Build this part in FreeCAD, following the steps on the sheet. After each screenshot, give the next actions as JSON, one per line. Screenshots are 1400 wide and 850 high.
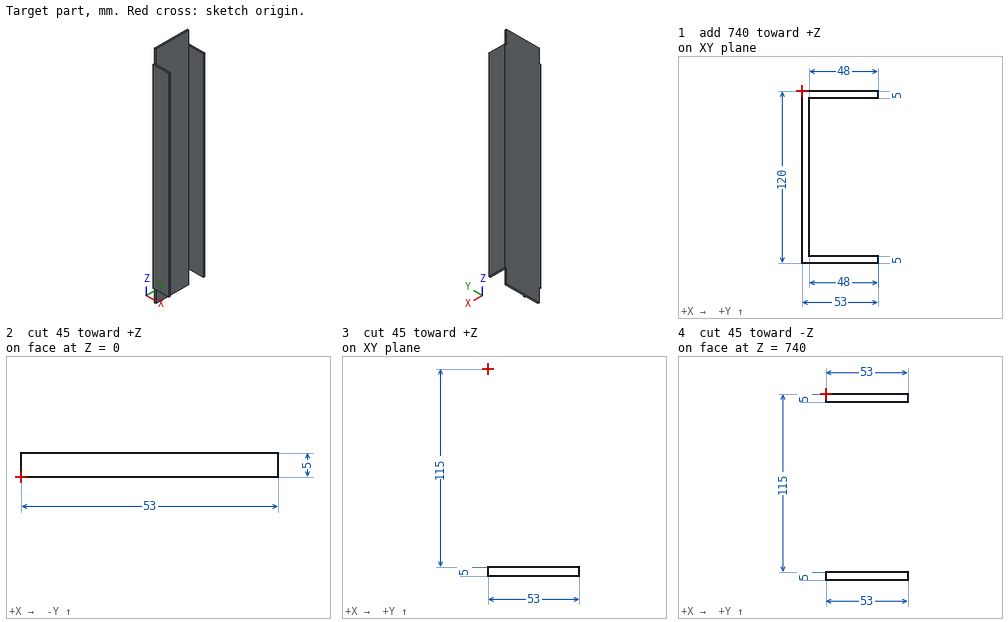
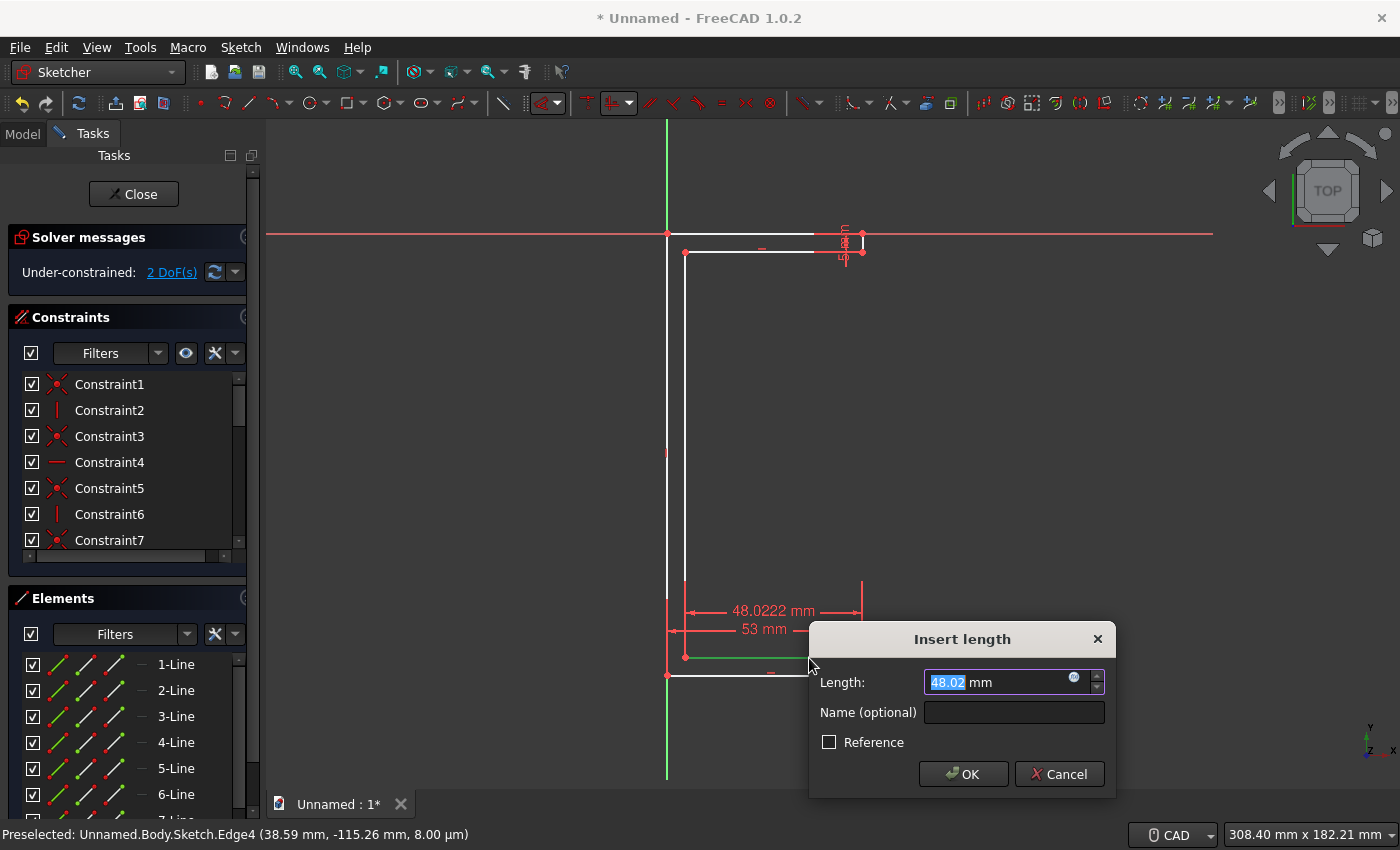
{"action": "type", "text": "48"}
{"action": "key", "text": "Return"}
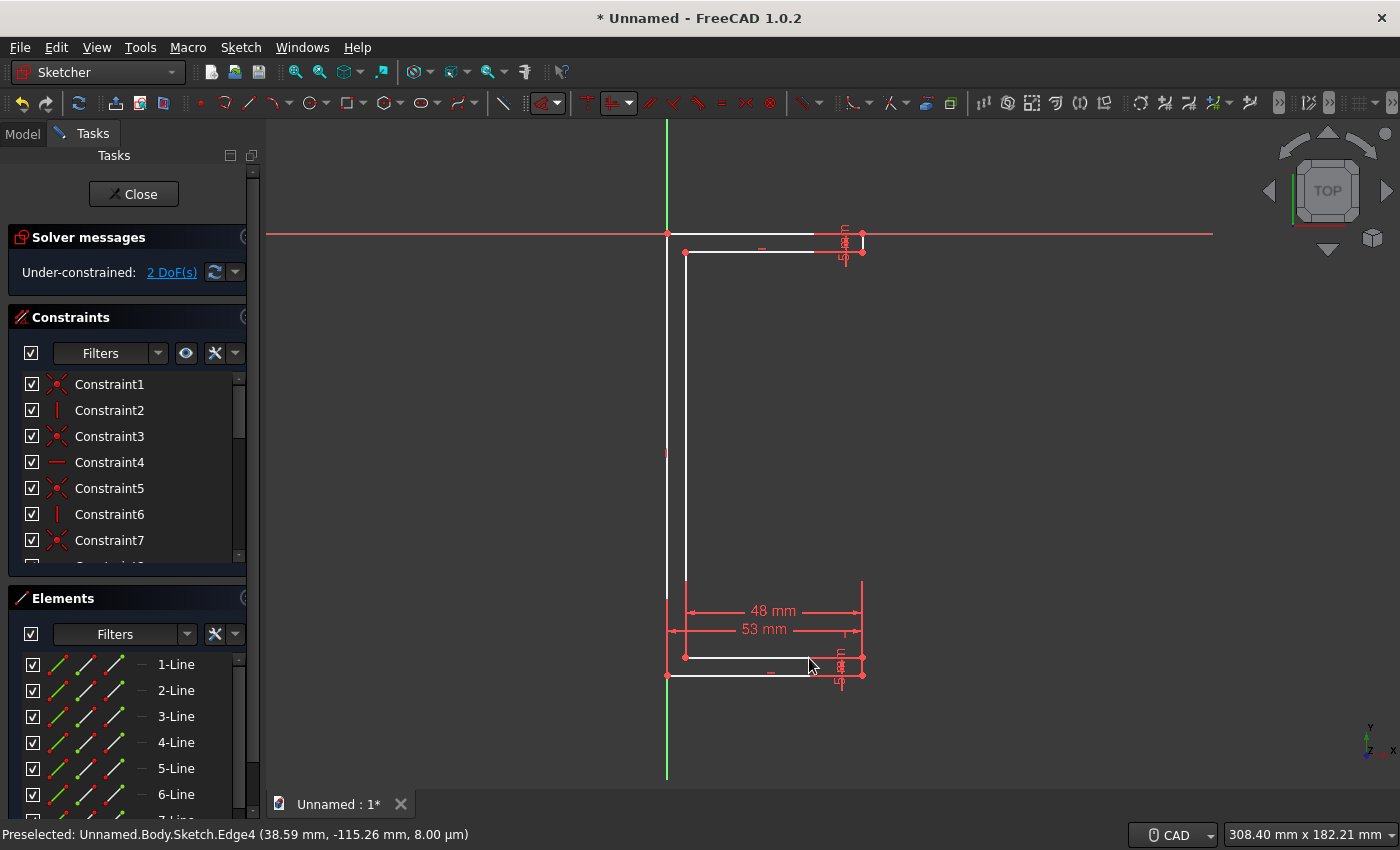
{"action": "left_click", "coordinate": [739, 252]}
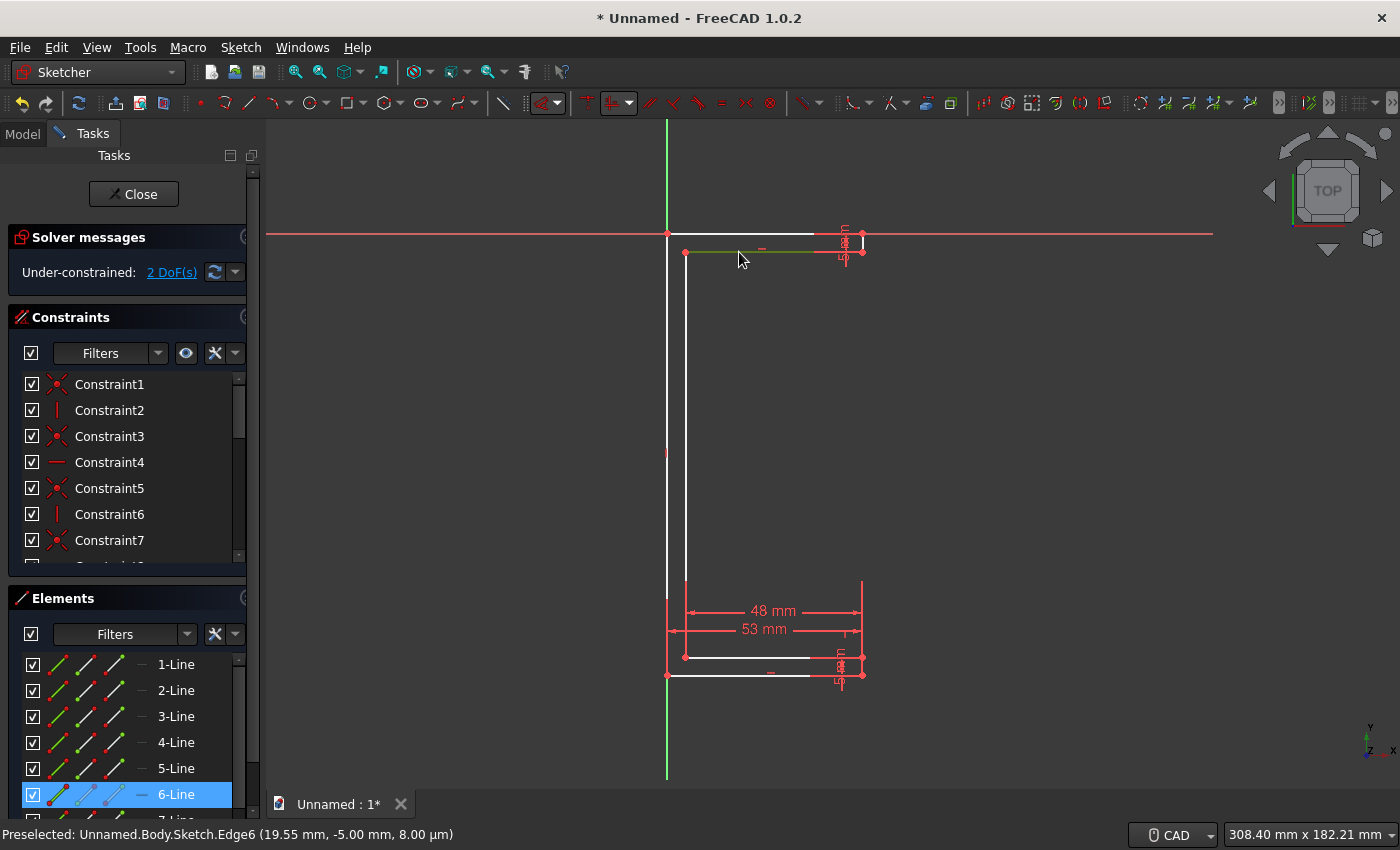
{"action": "key", "text": "l"}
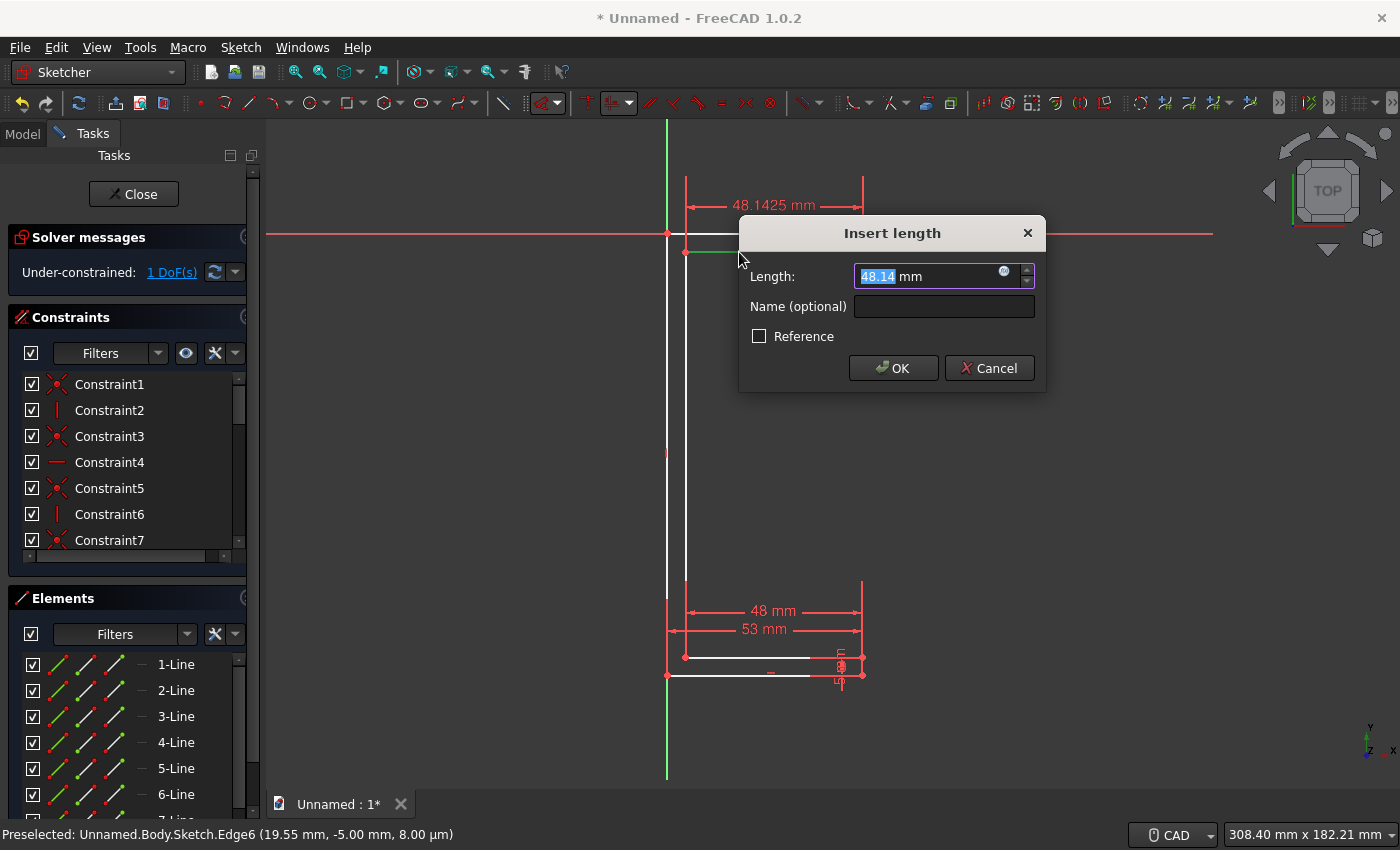
{"action": "type", "text": "48"}
{"action": "key", "text": "Return"}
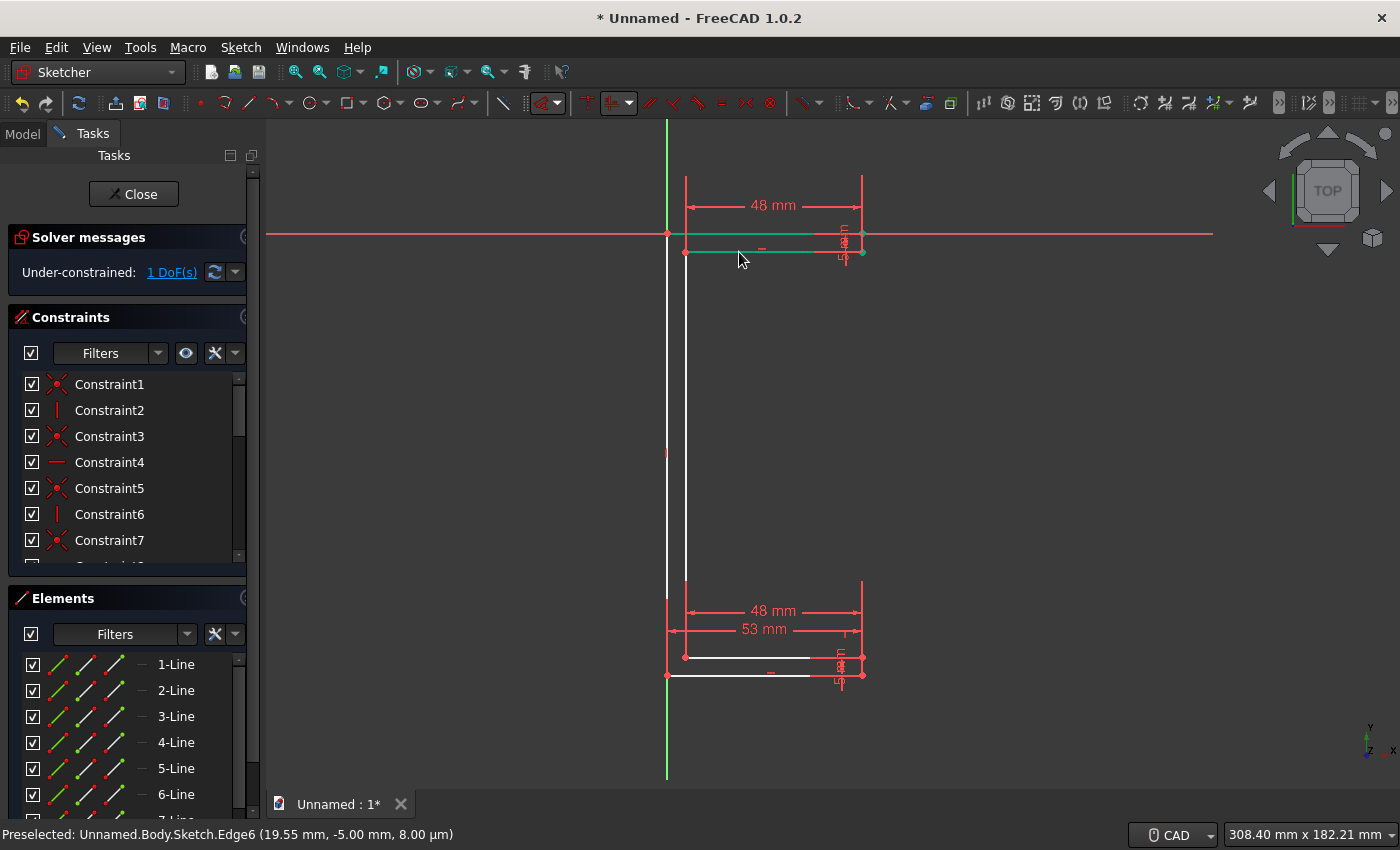
{"action": "left_click", "coordinate": [667, 366]}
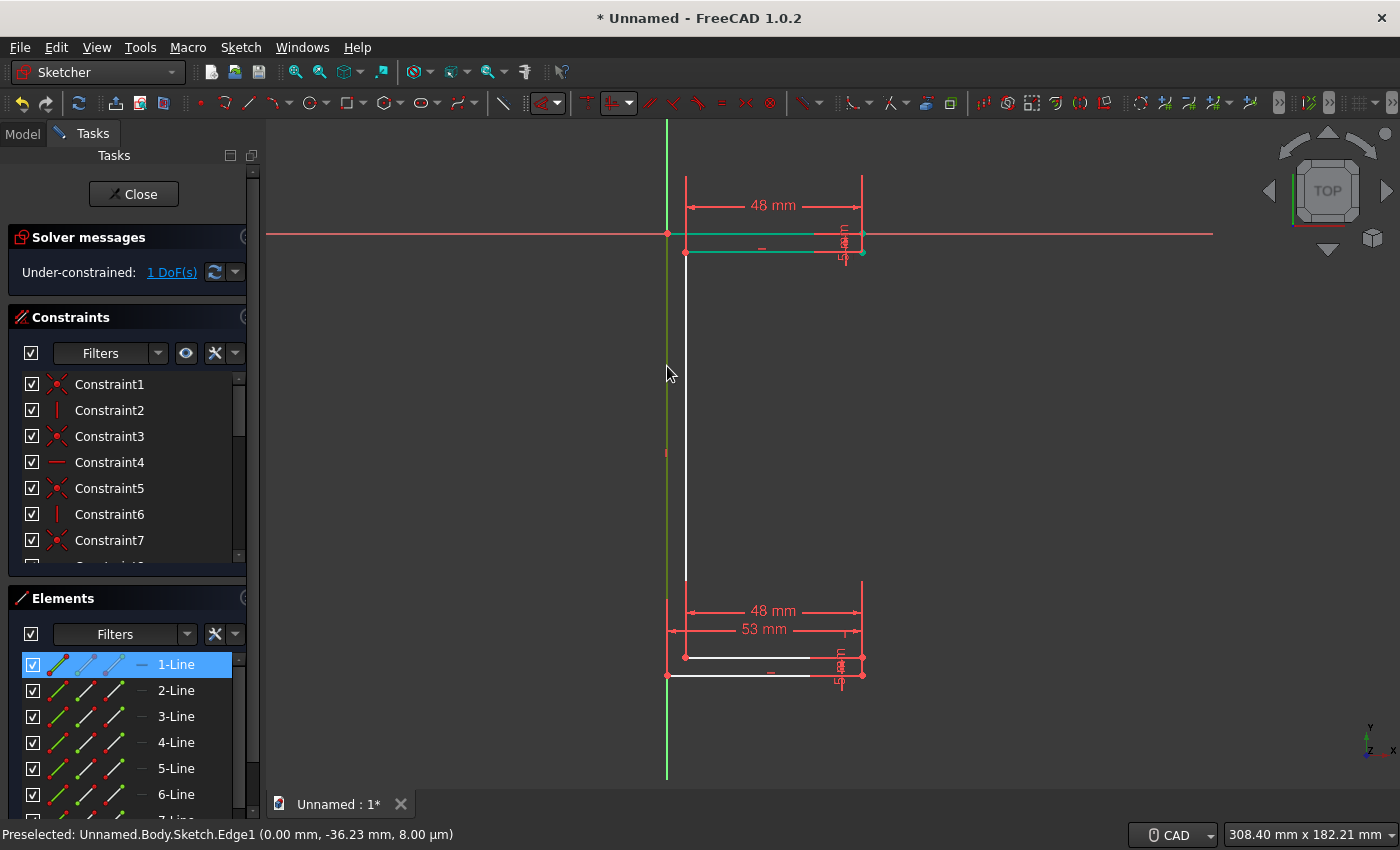
{"action": "key", "text": "i"}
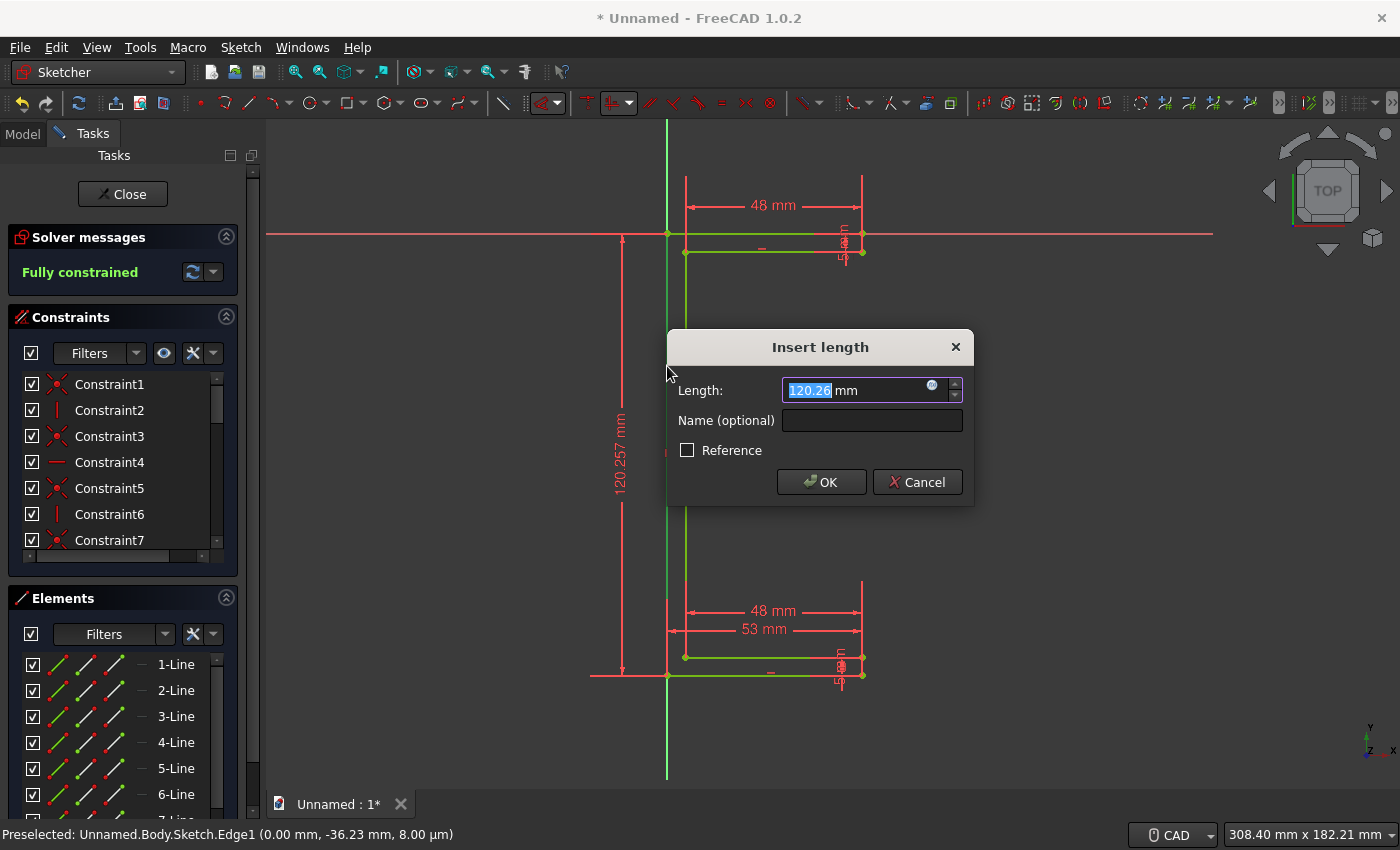
{"action": "type", "text": "120"}
{"action": "key", "text": "Return"}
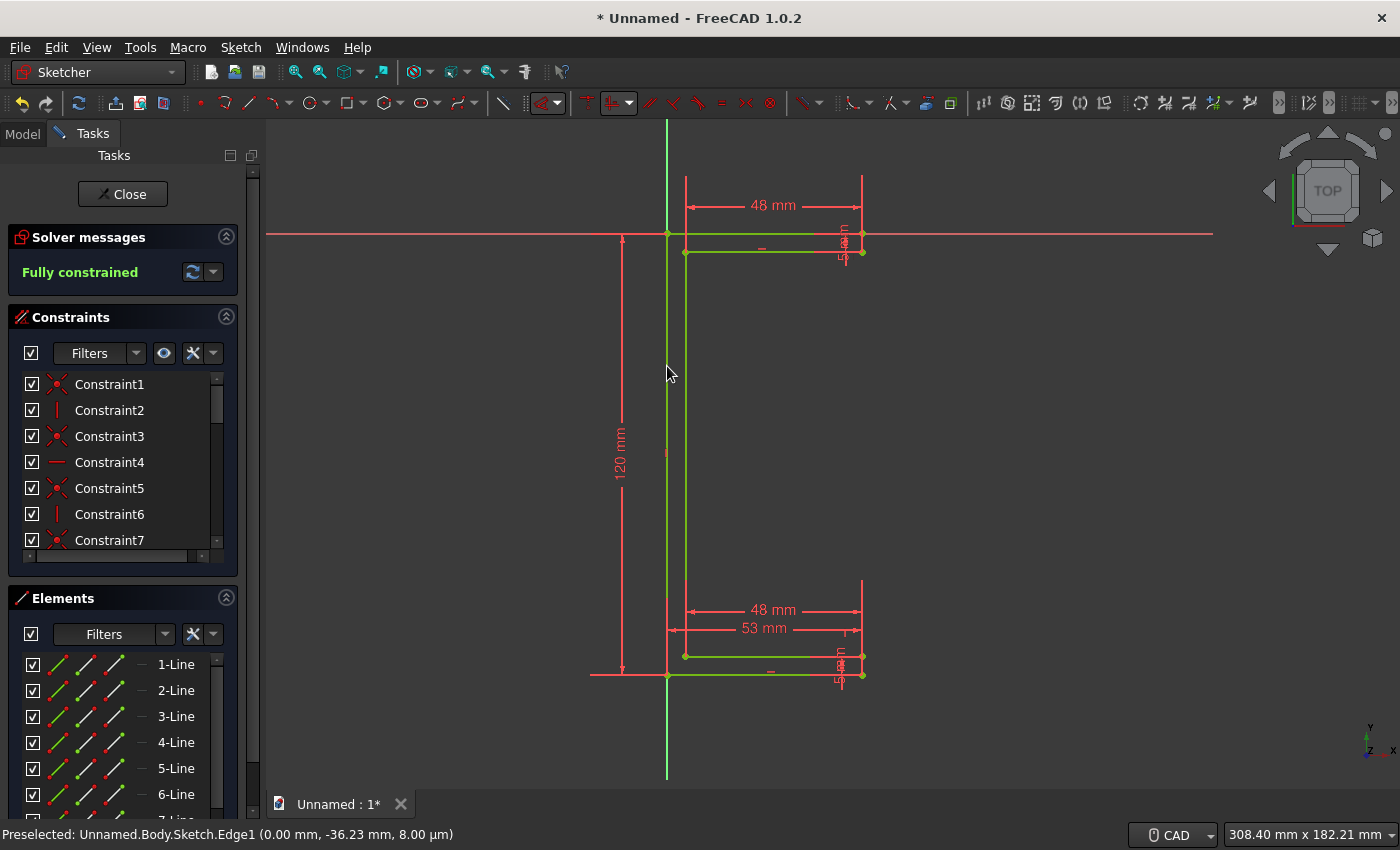
{"action": "left_click", "coordinate": [123, 194]}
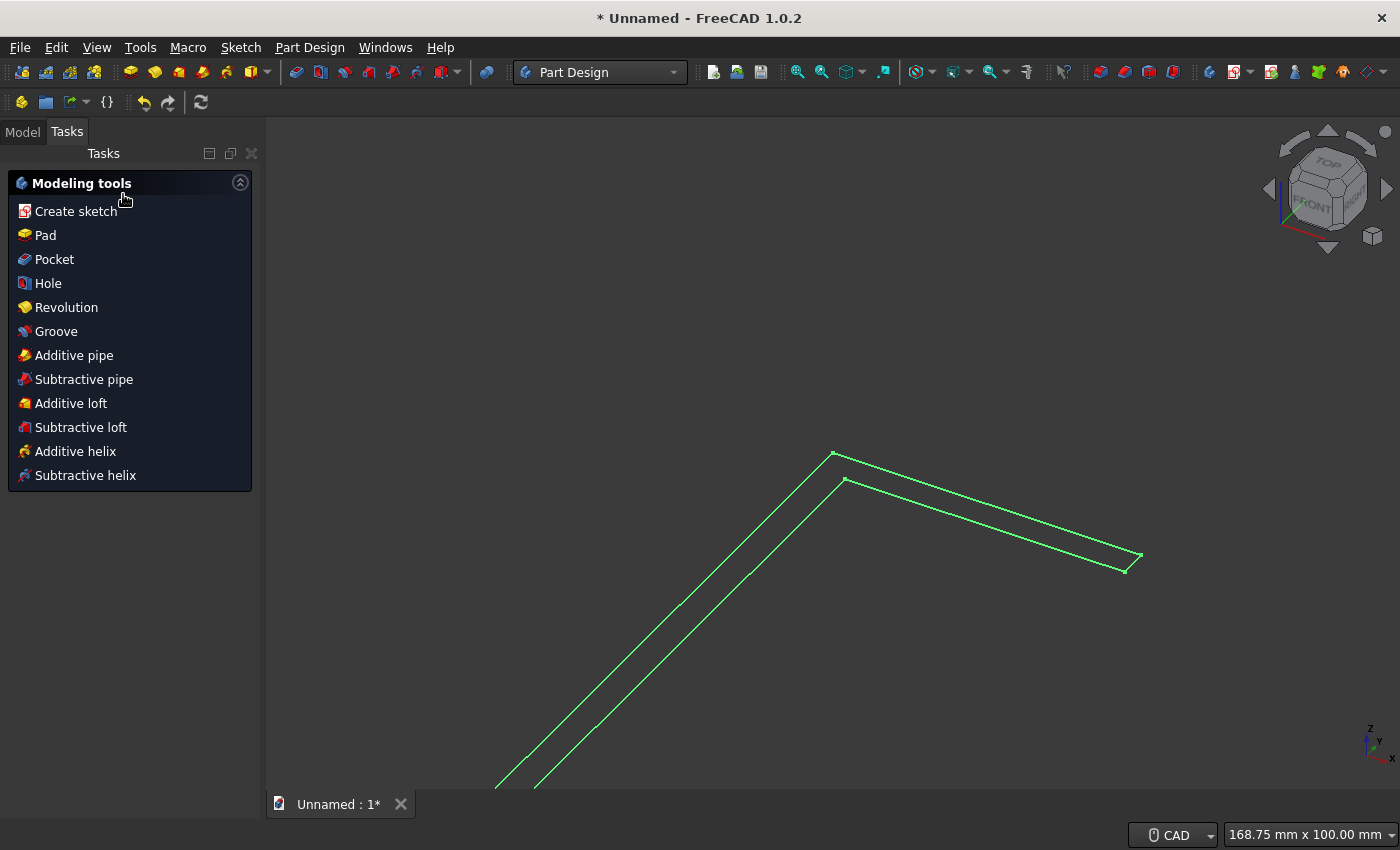
{"action": "left_click", "coordinate": [132, 72]}